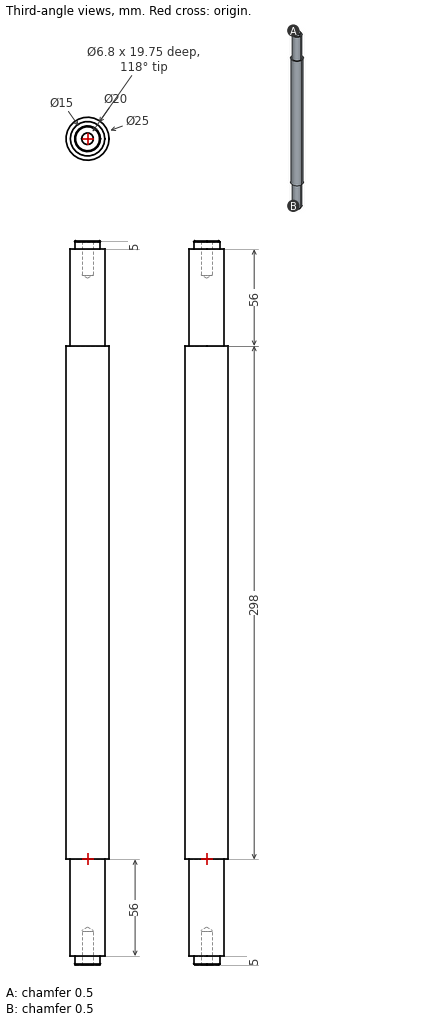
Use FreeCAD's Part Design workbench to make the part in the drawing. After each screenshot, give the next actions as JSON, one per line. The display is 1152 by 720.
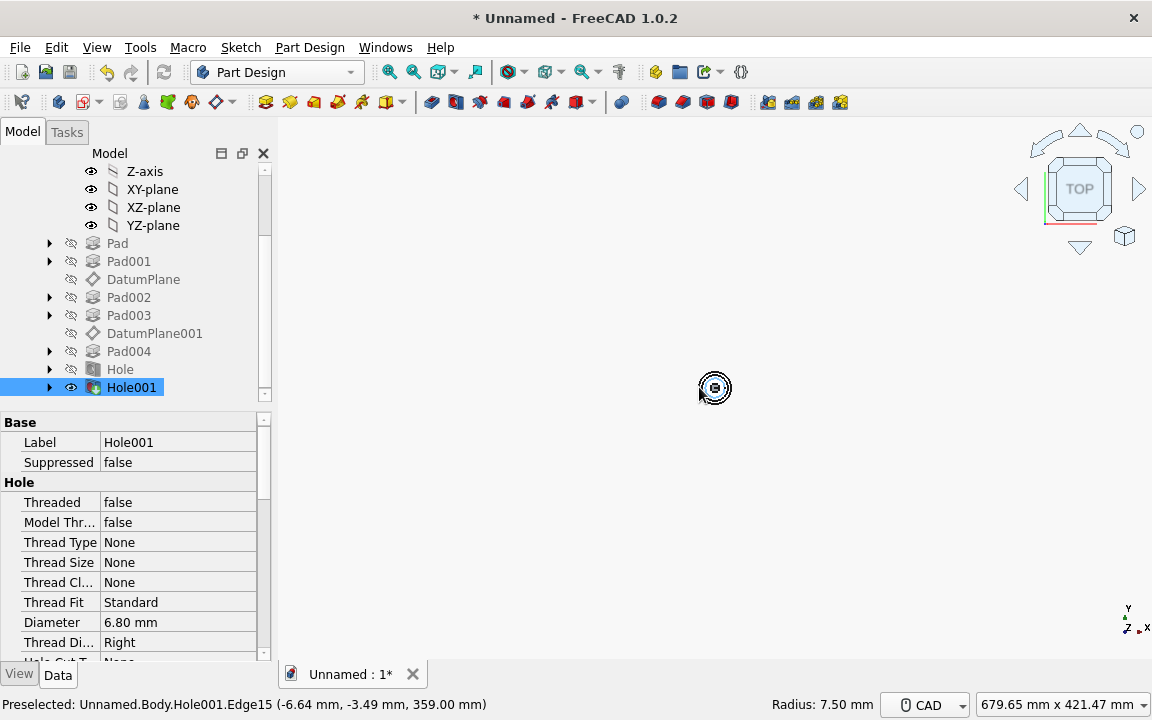
{"action": "left_click", "coordinate": [684, 102]}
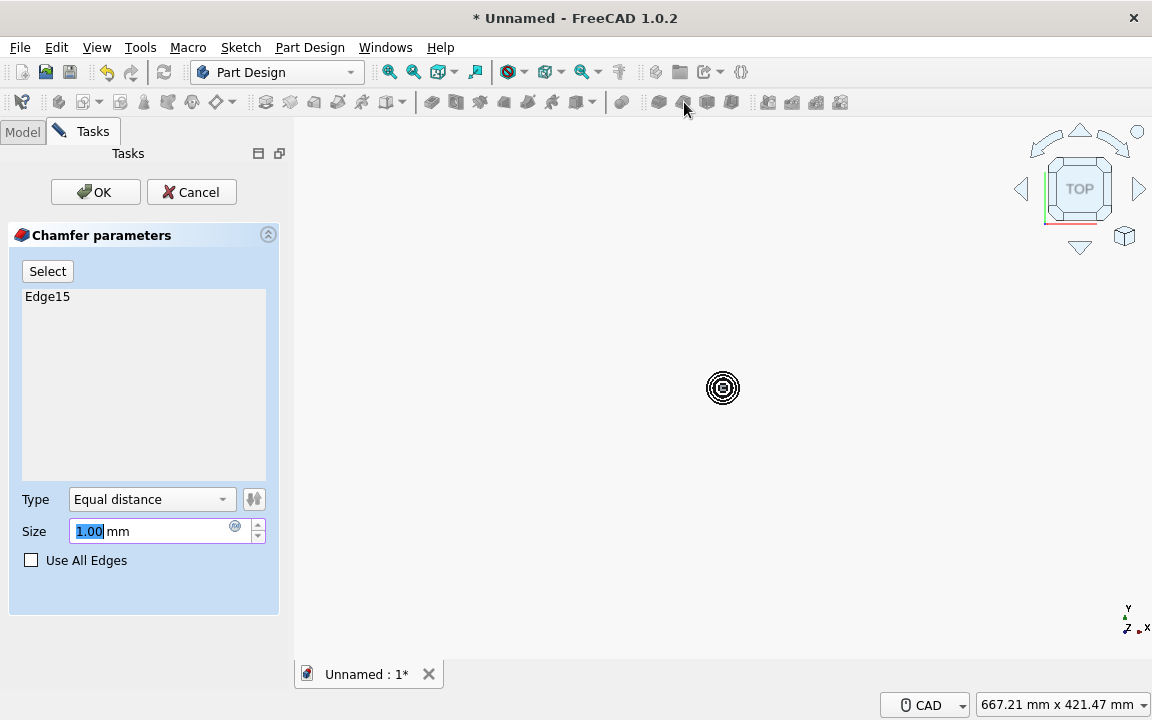
{"action": "type", "text": "0.5"}
{"action": "key", "text": "Tab"}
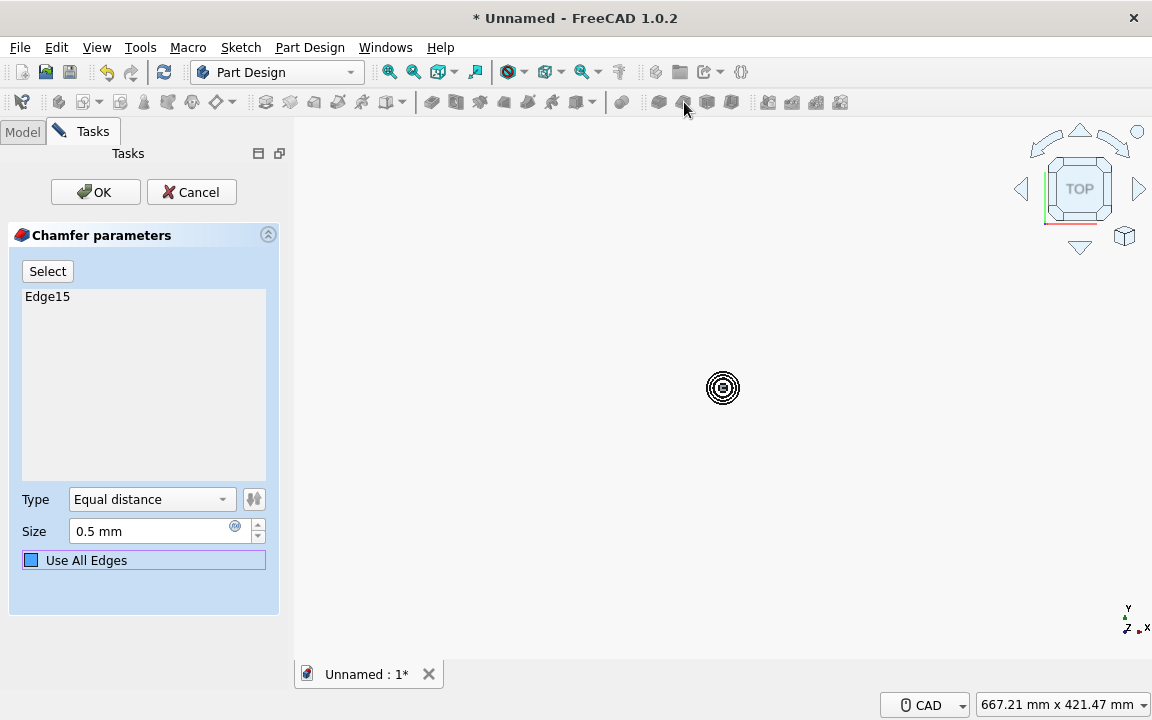
{"action": "left_click", "coordinate": [96, 192]}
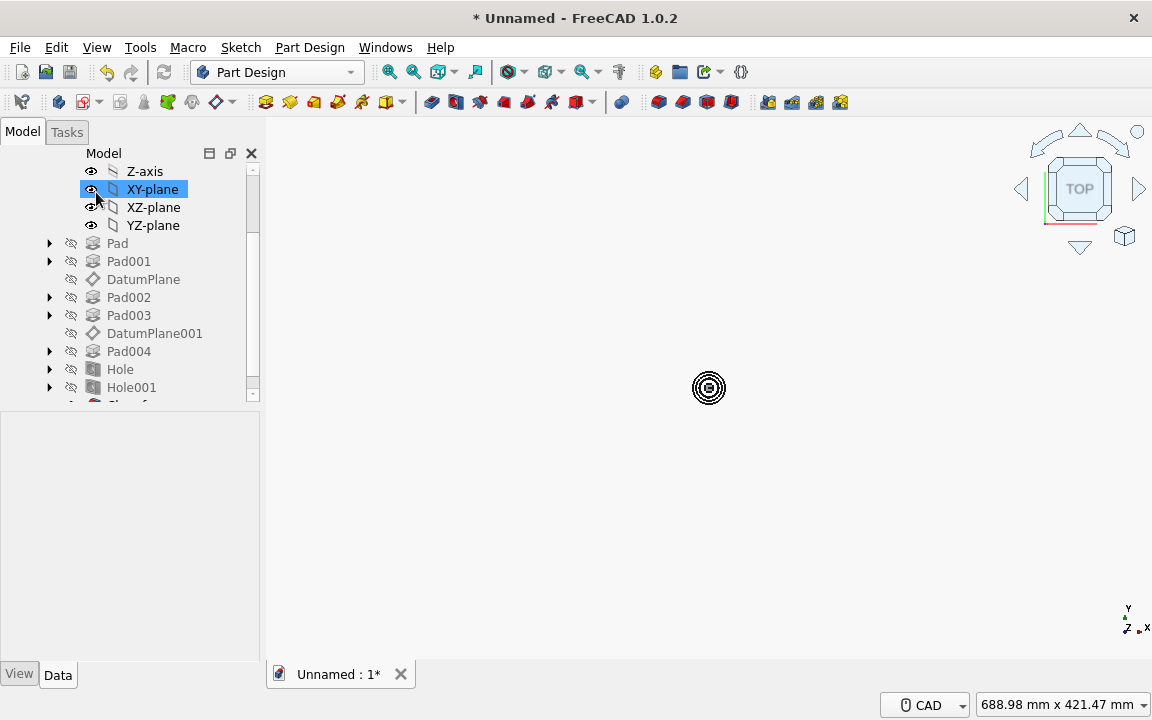
{"action": "left_click", "coordinate": [390, 72]}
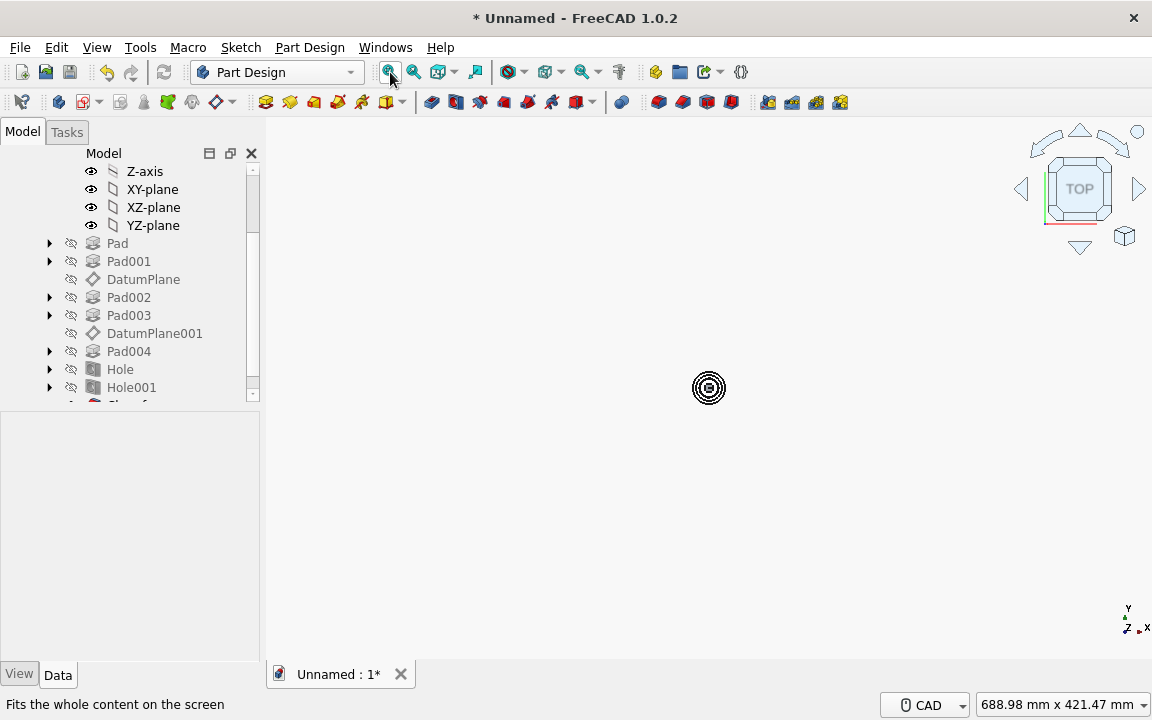
{"action": "key", "text": "0"}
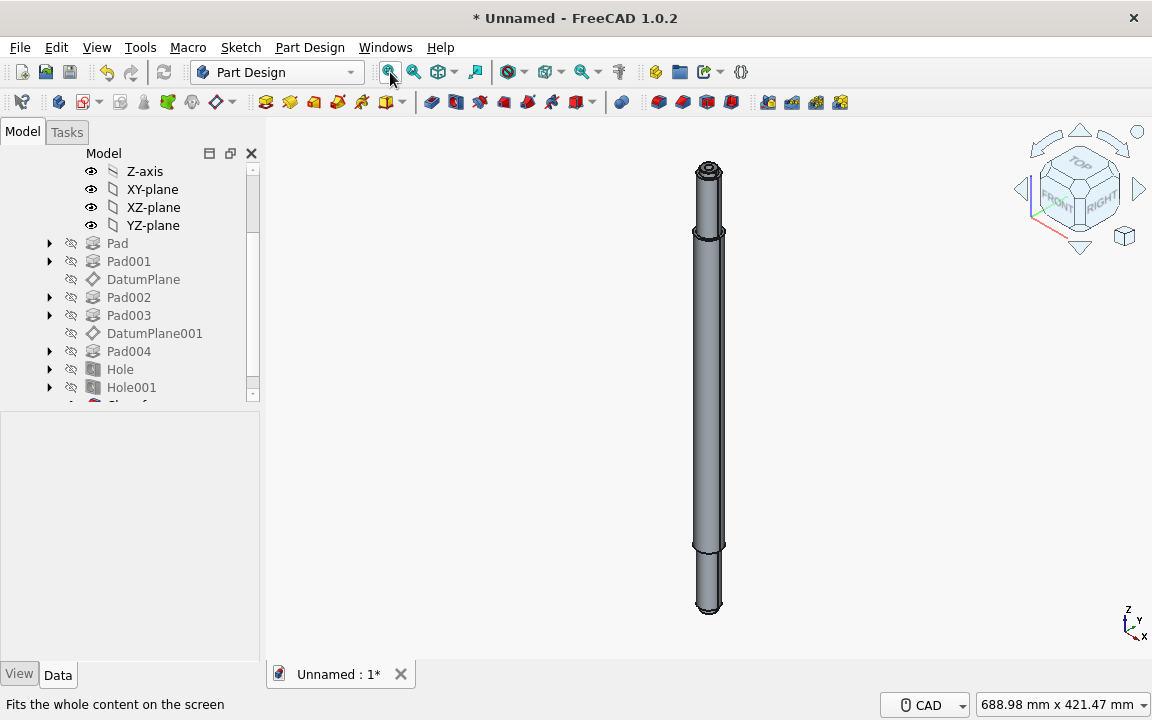
{"action": "key", "text": "2"}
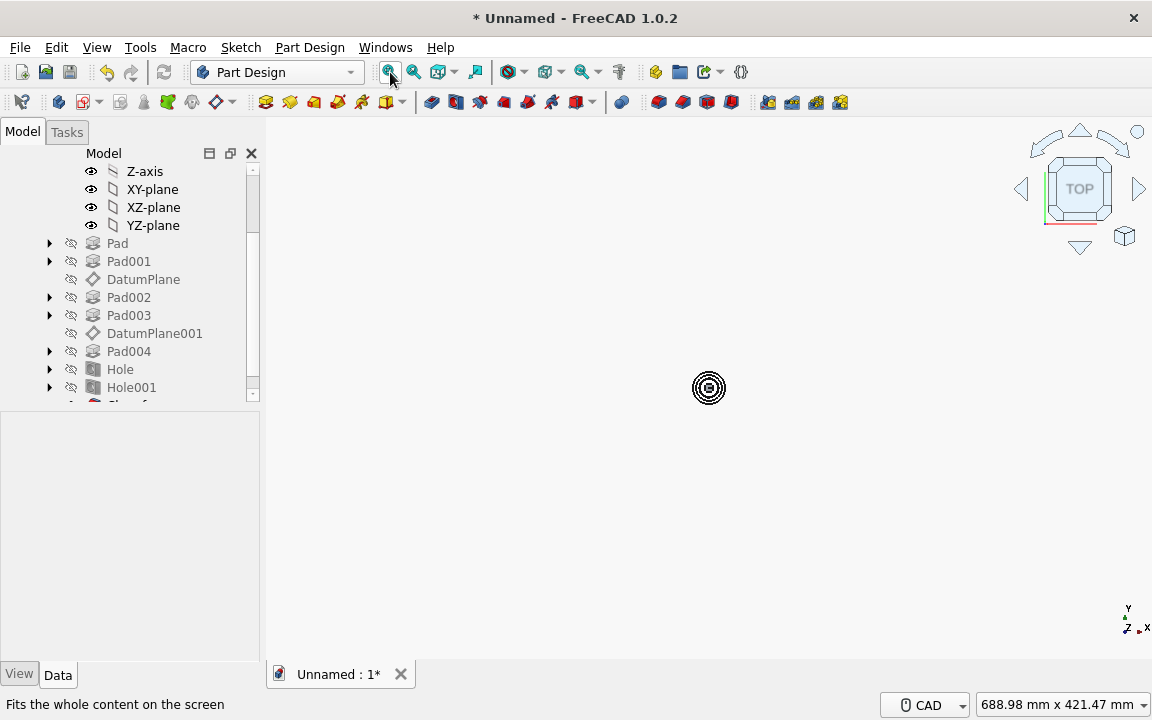
{"action": "left_click", "coordinate": [390, 72]}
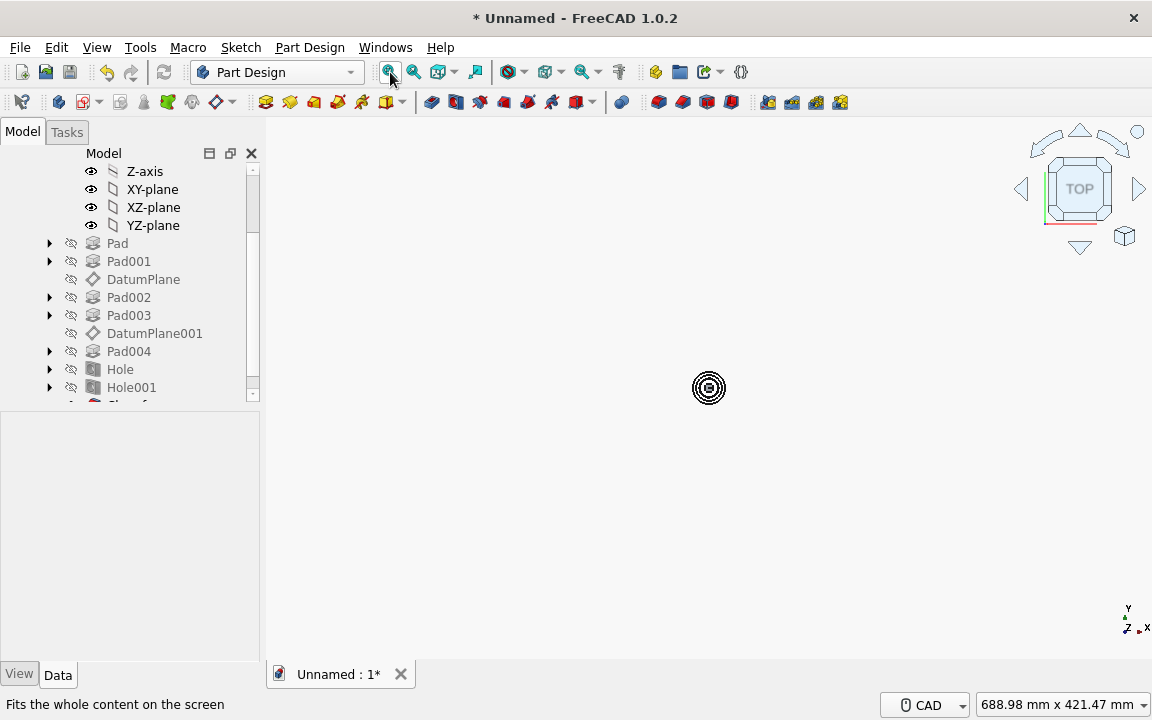
{"action": "key", "text": "1"}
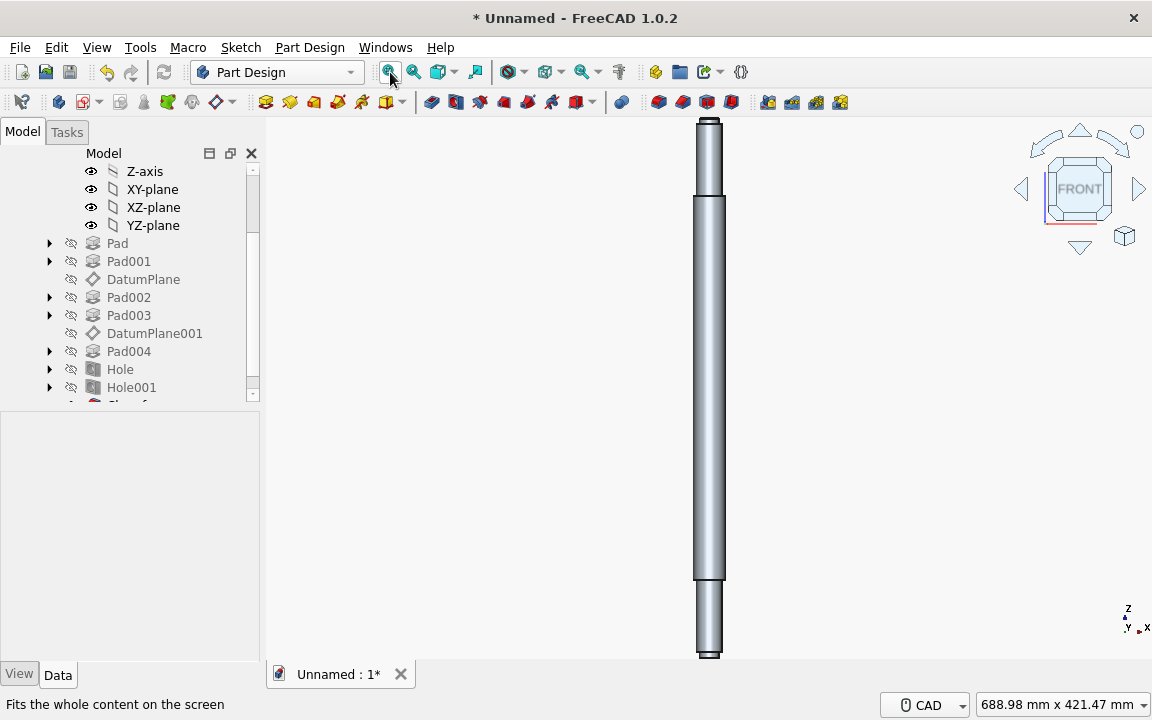
{"action": "key", "text": "3"}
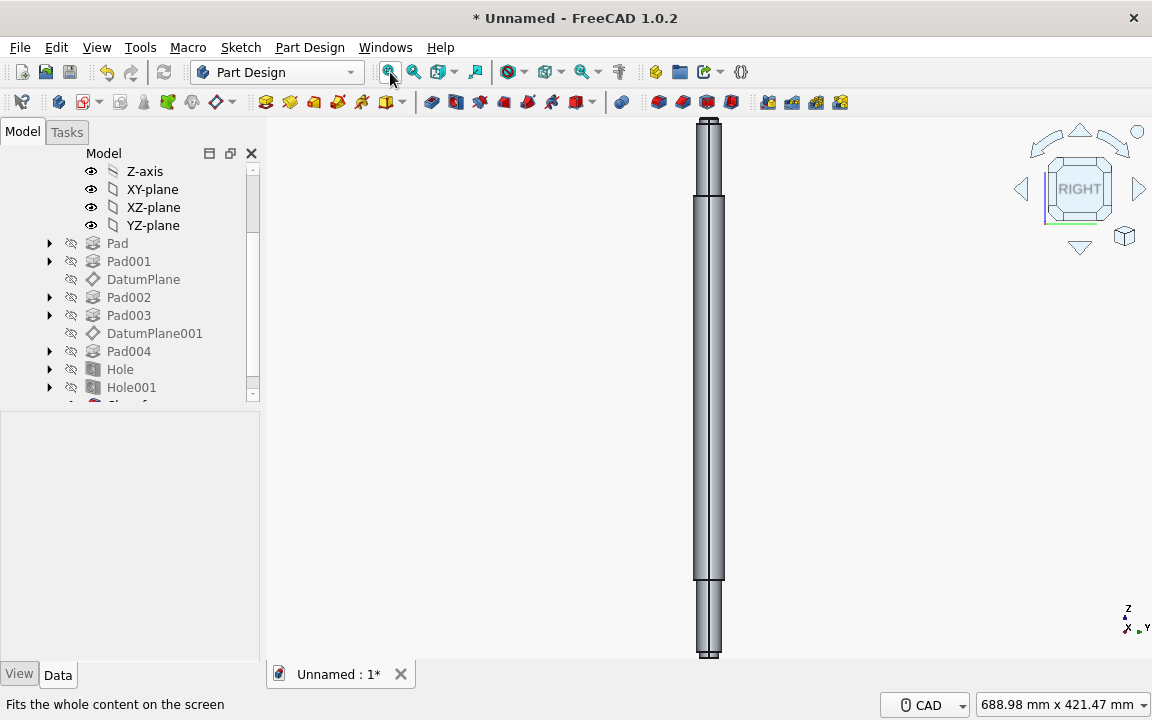
{"action": "key", "text": "5"}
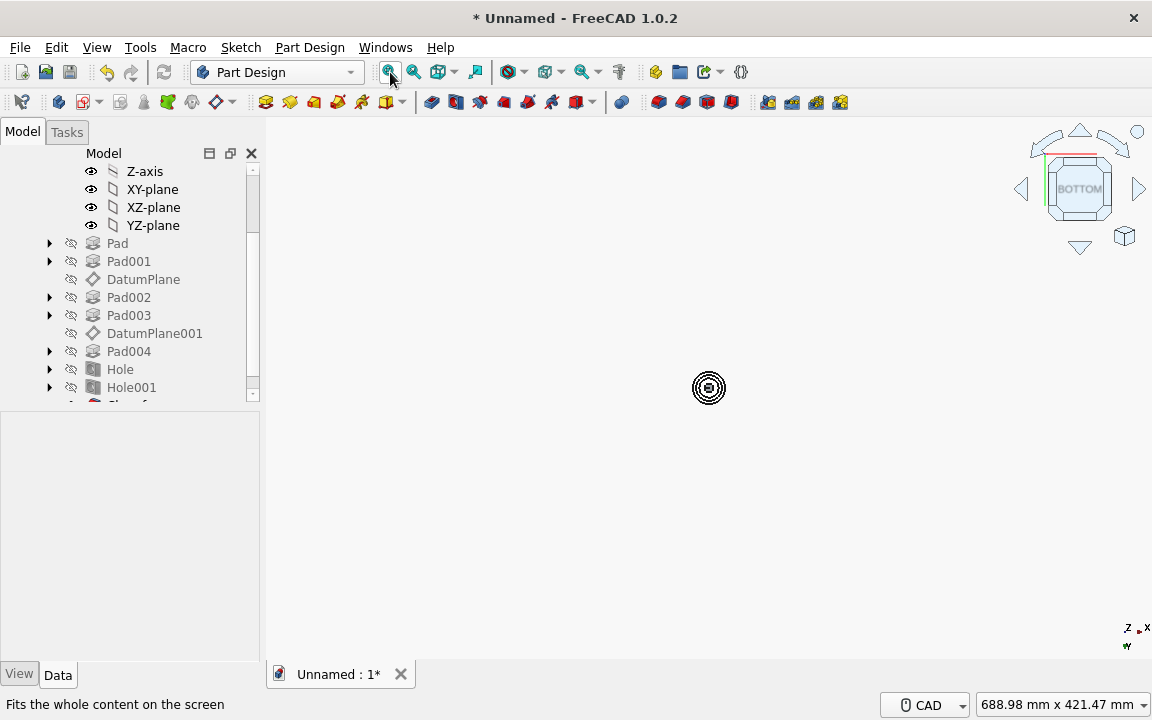
{"action": "left_click", "coordinate": [390, 72]}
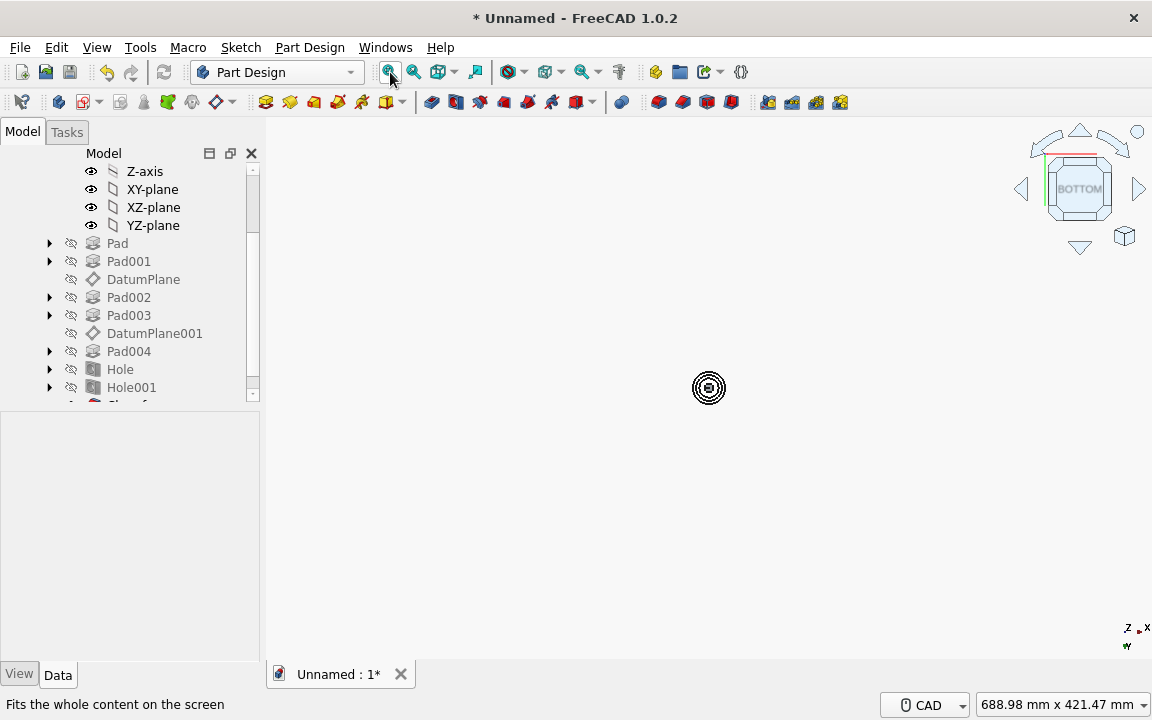
{"action": "left_click", "coordinate": [701, 393]}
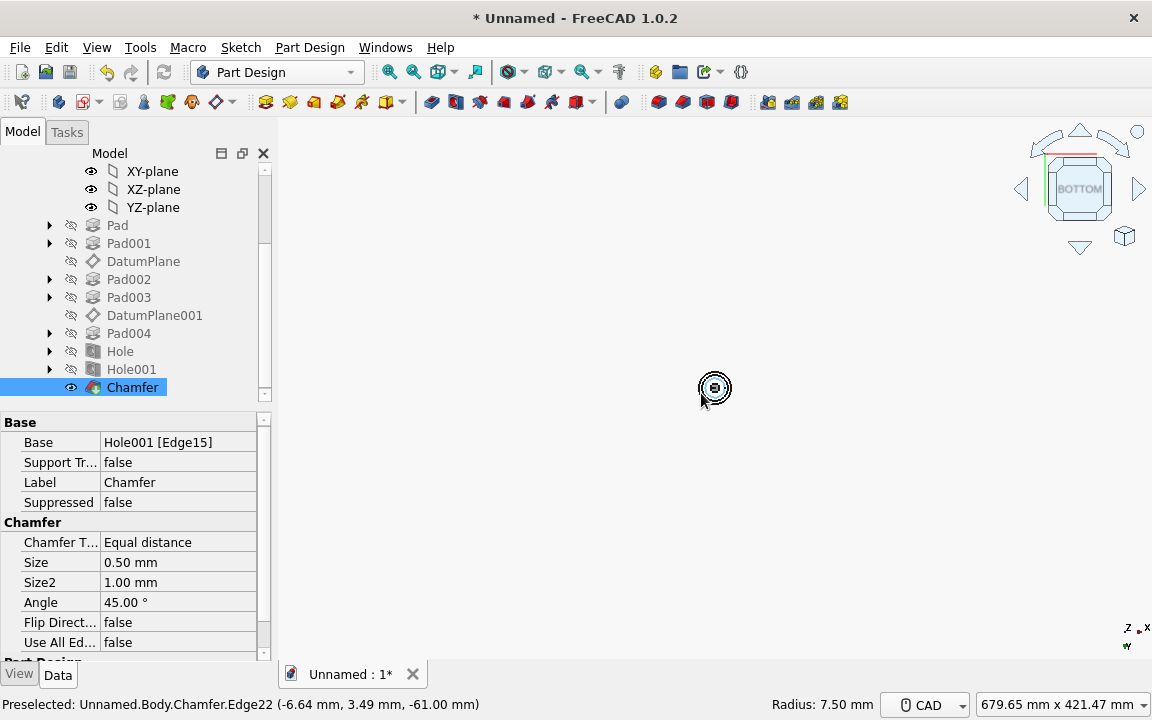
{"action": "left_click", "coordinate": [684, 102]}